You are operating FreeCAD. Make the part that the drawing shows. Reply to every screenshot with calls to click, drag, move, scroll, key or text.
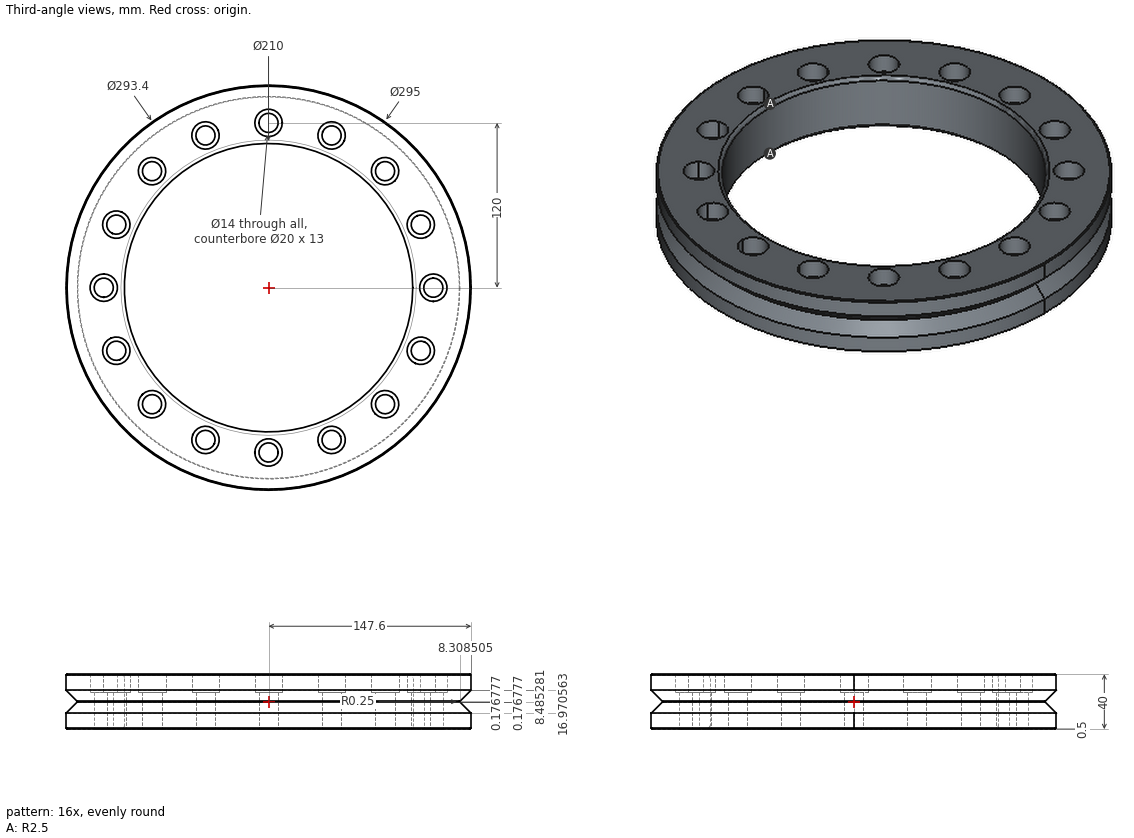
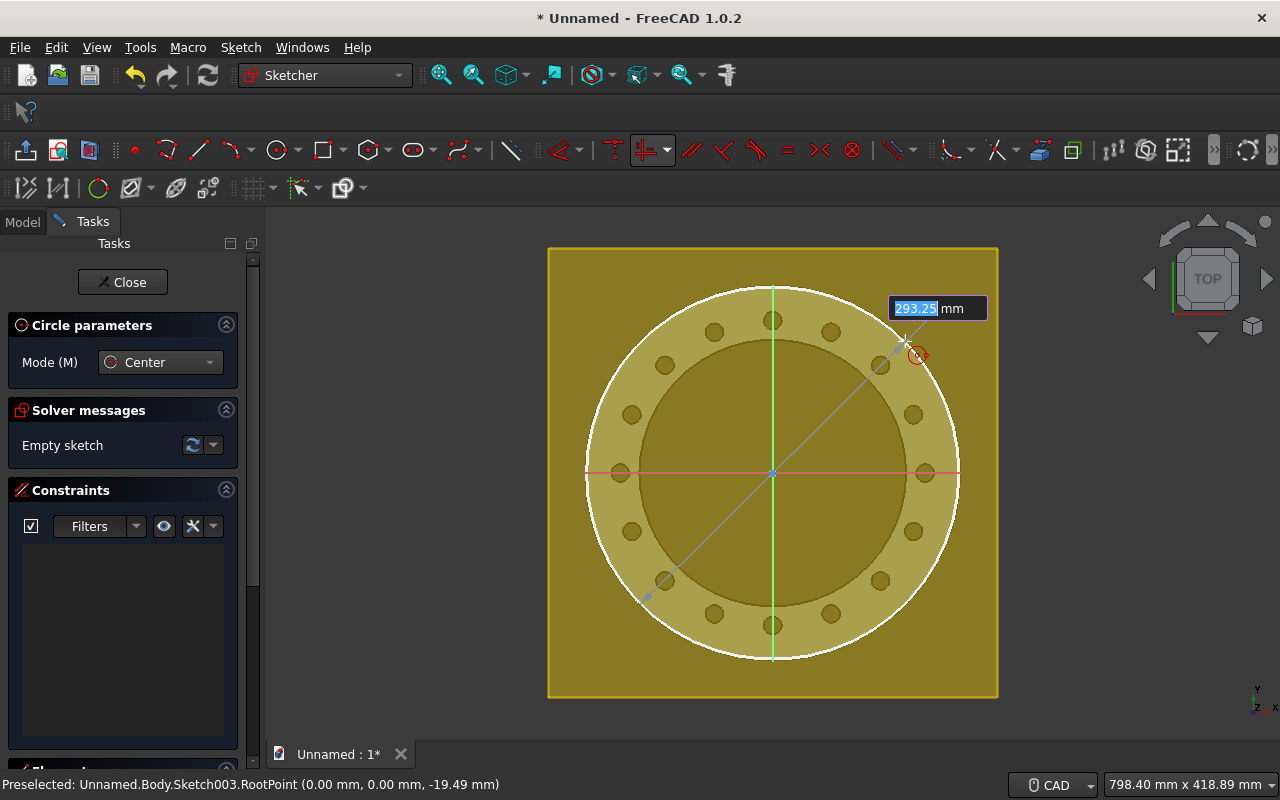
text(295)
key(Return)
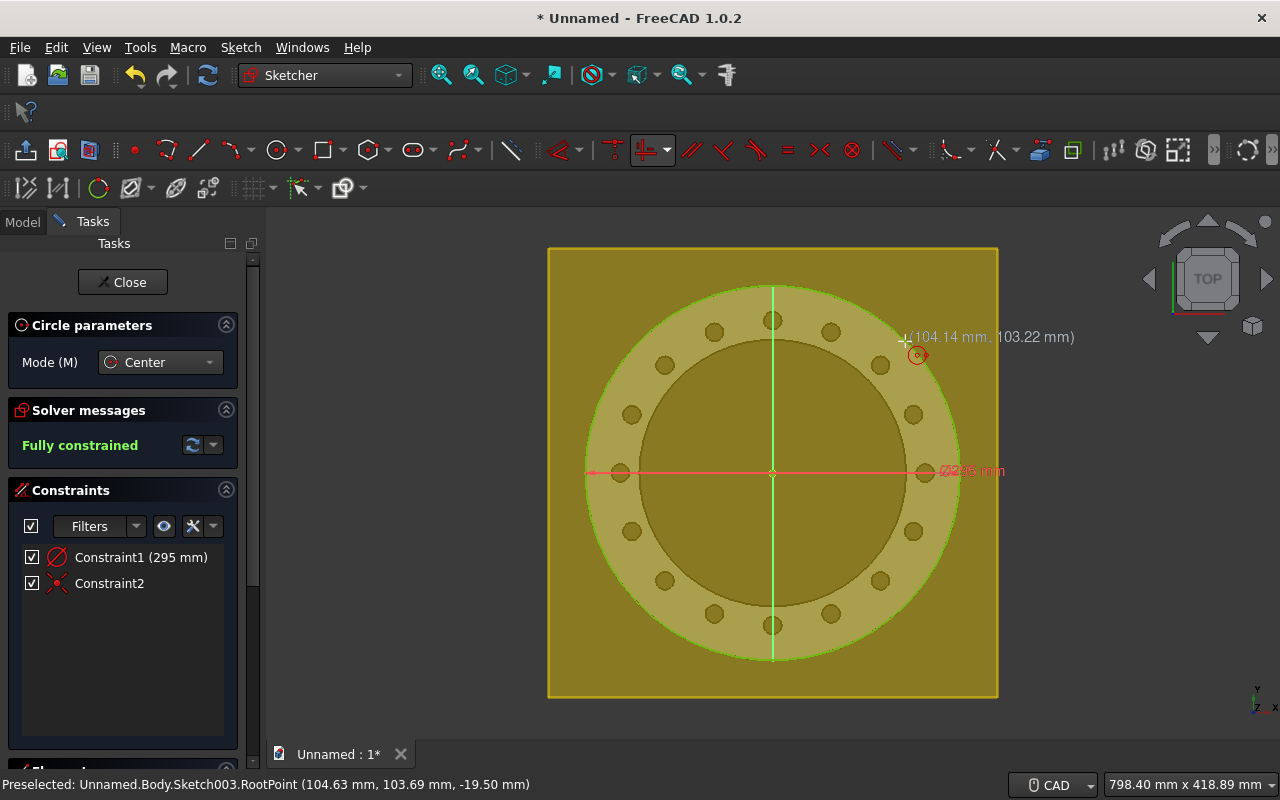
click(773, 473)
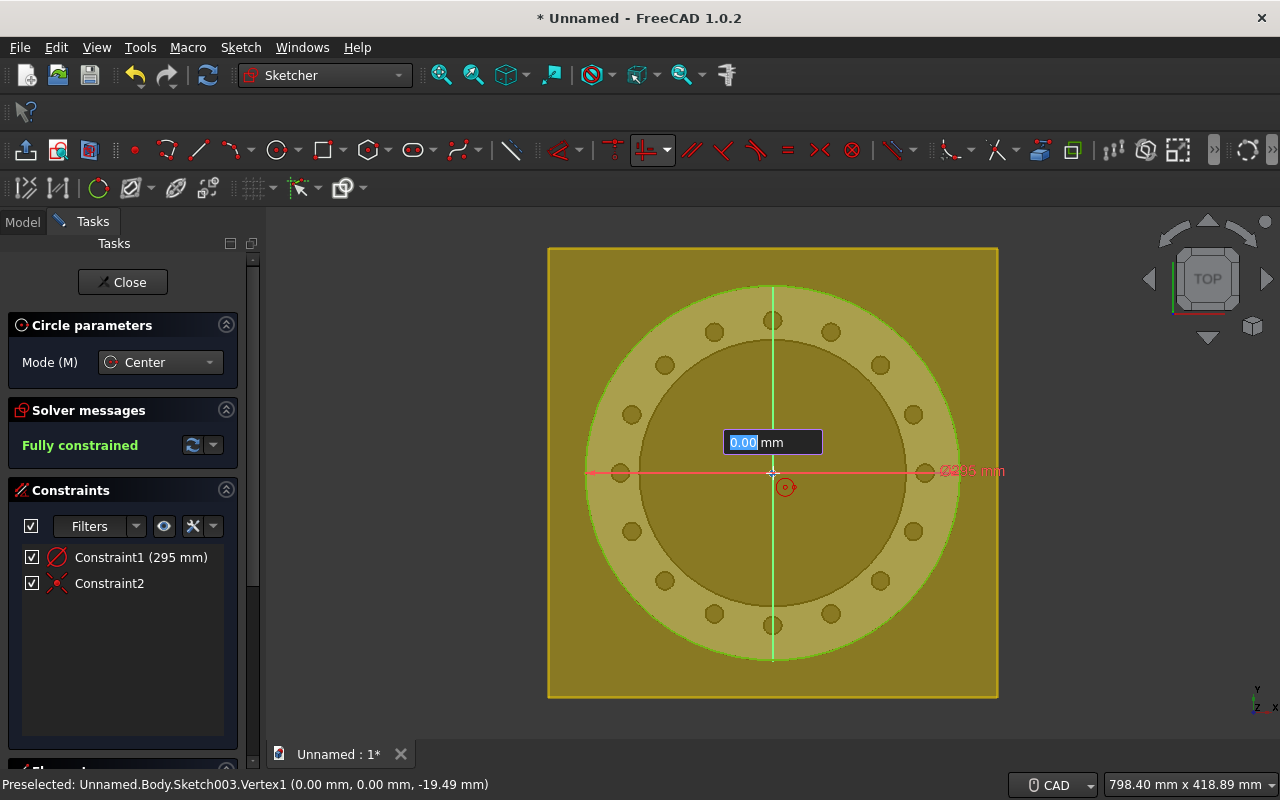
scroll(904, 341, up, 14)
move(902, 343)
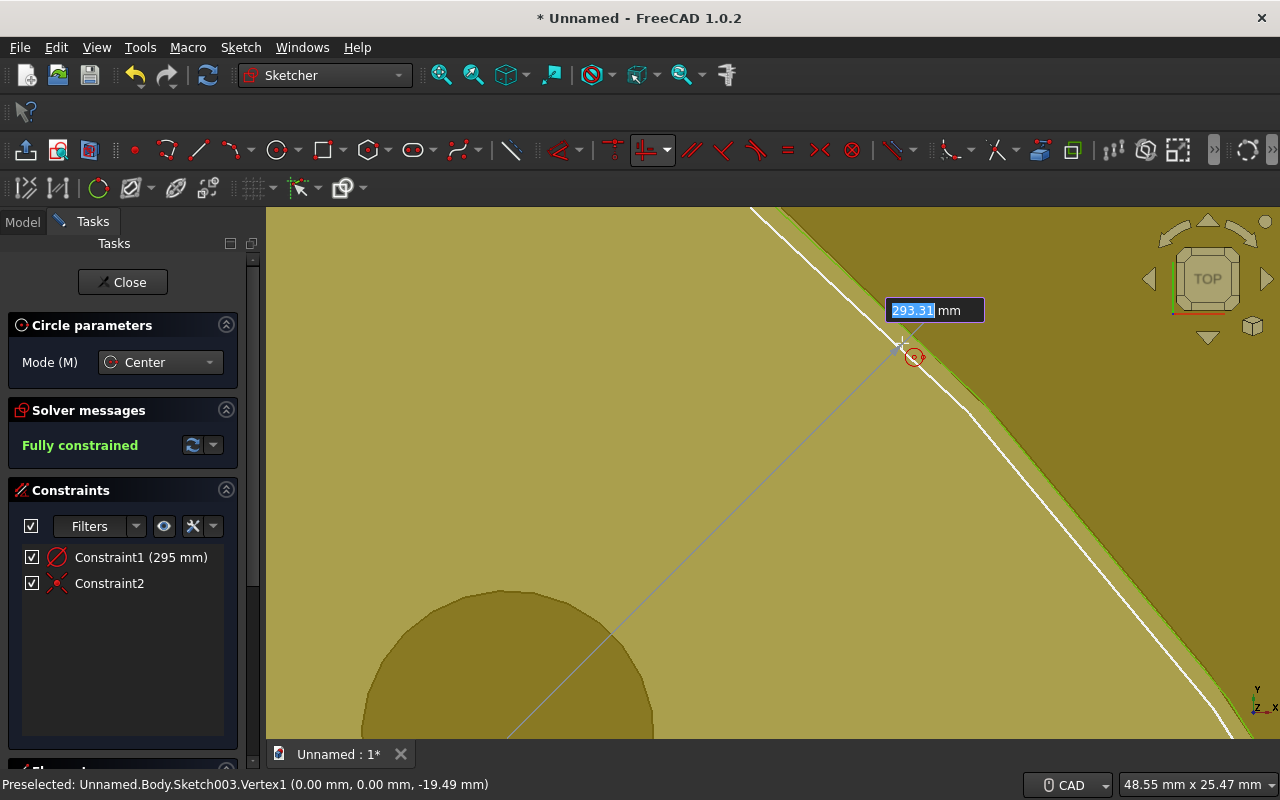
text(293.4)
key(Return)
key(Escape)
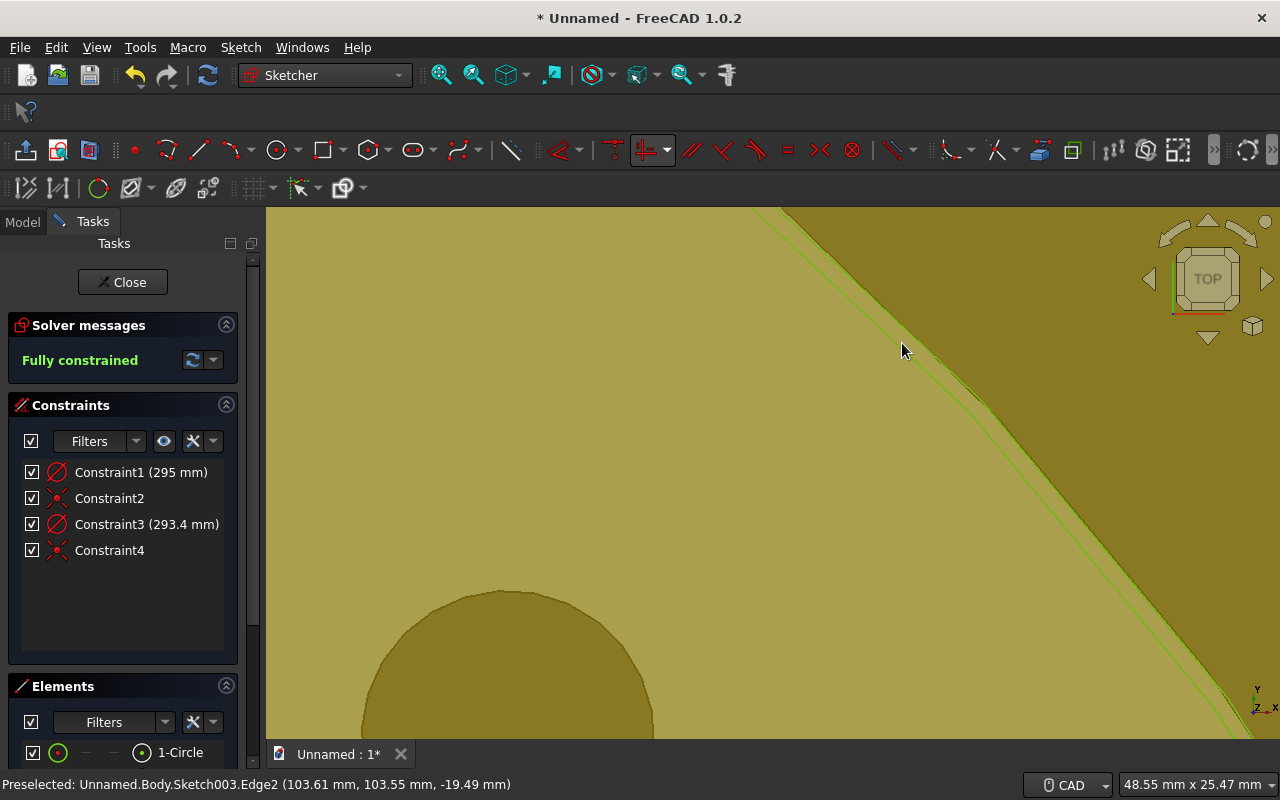
click(123, 282)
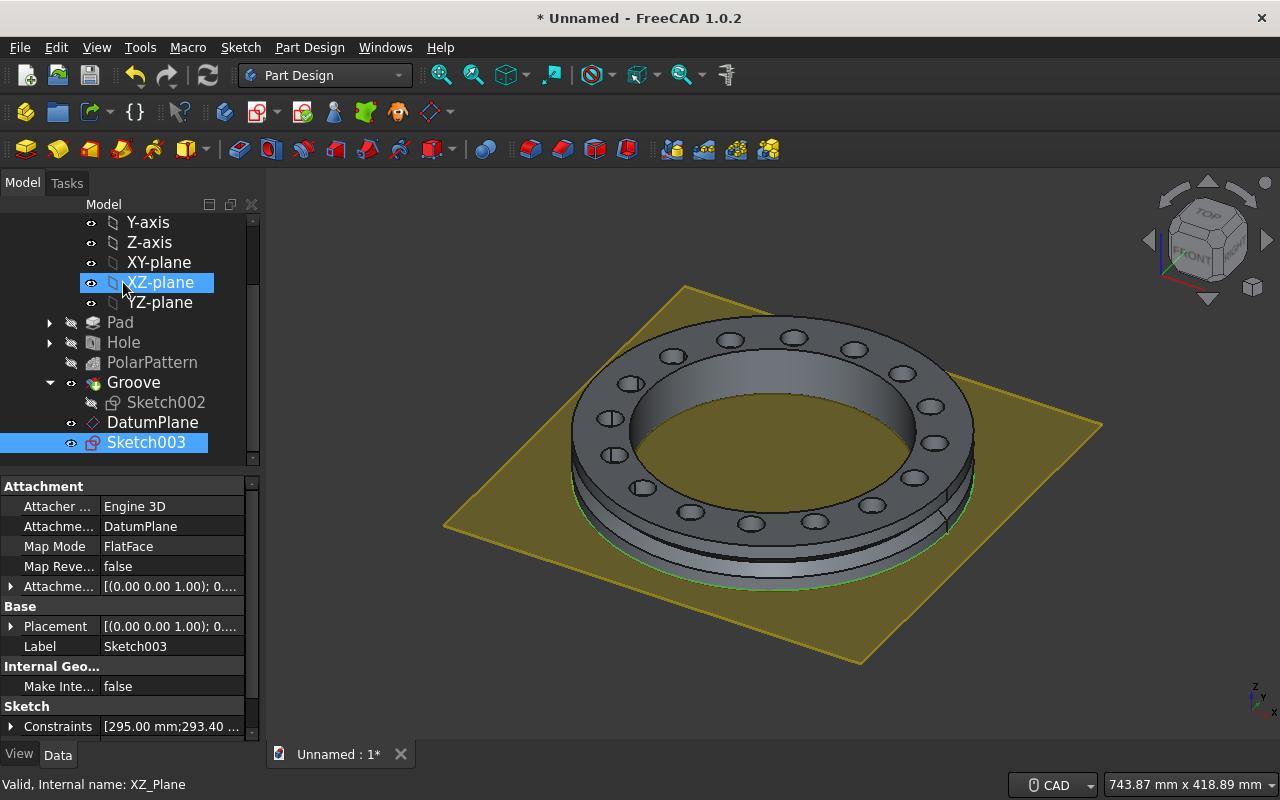
click(240, 150)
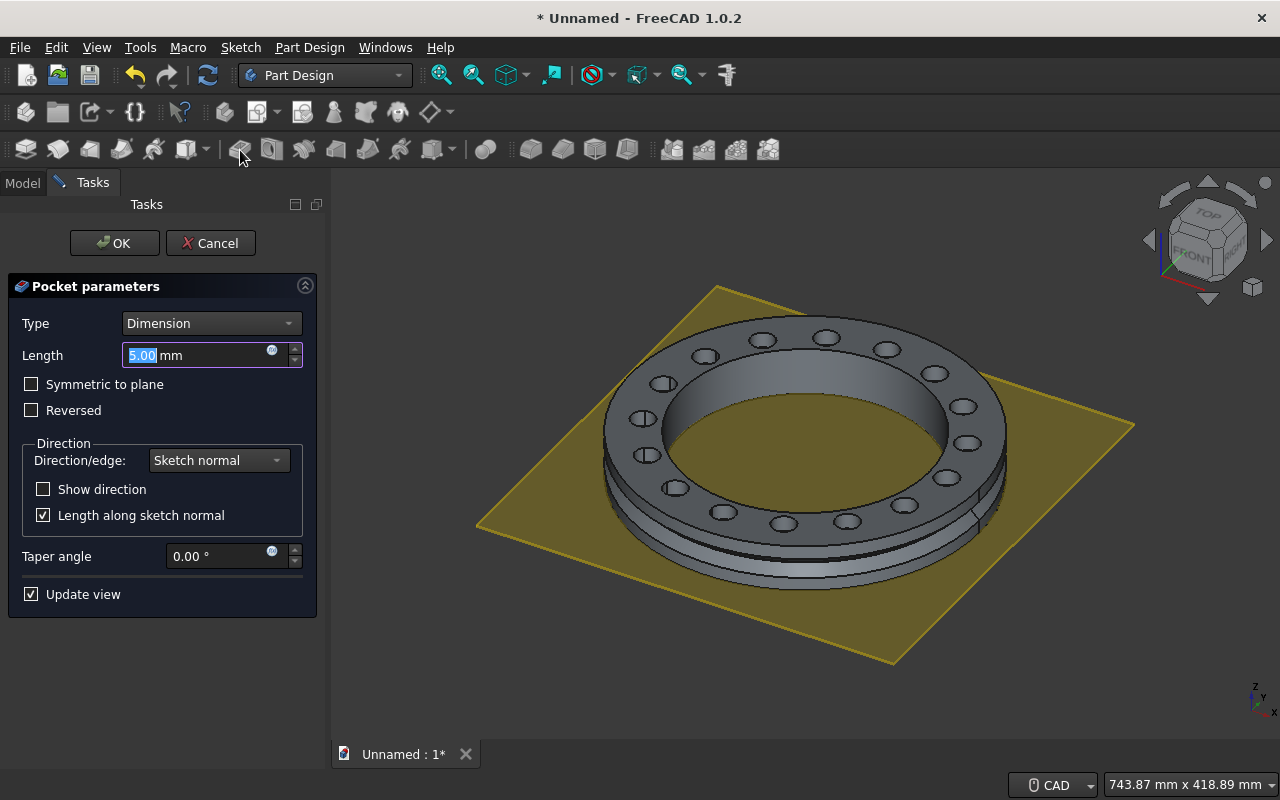
text(0.5)
key(Tab)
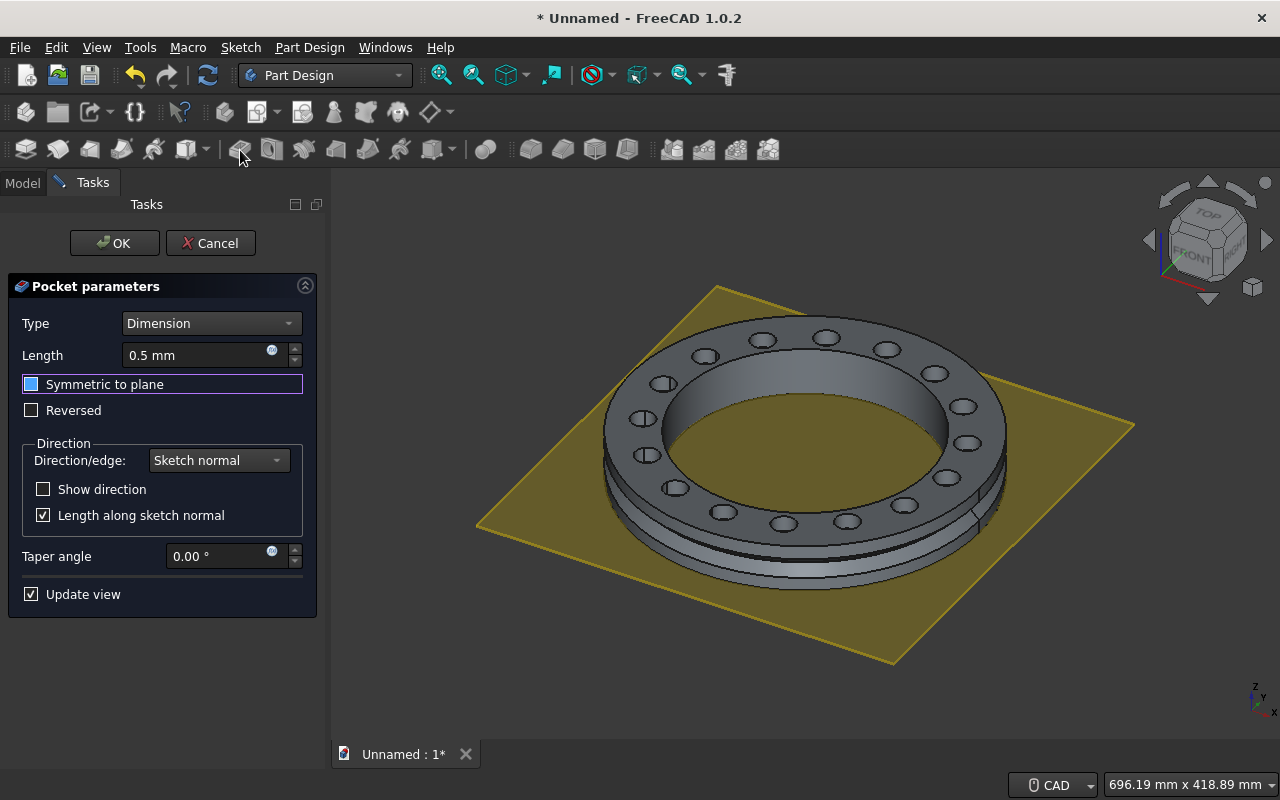
click(115, 243)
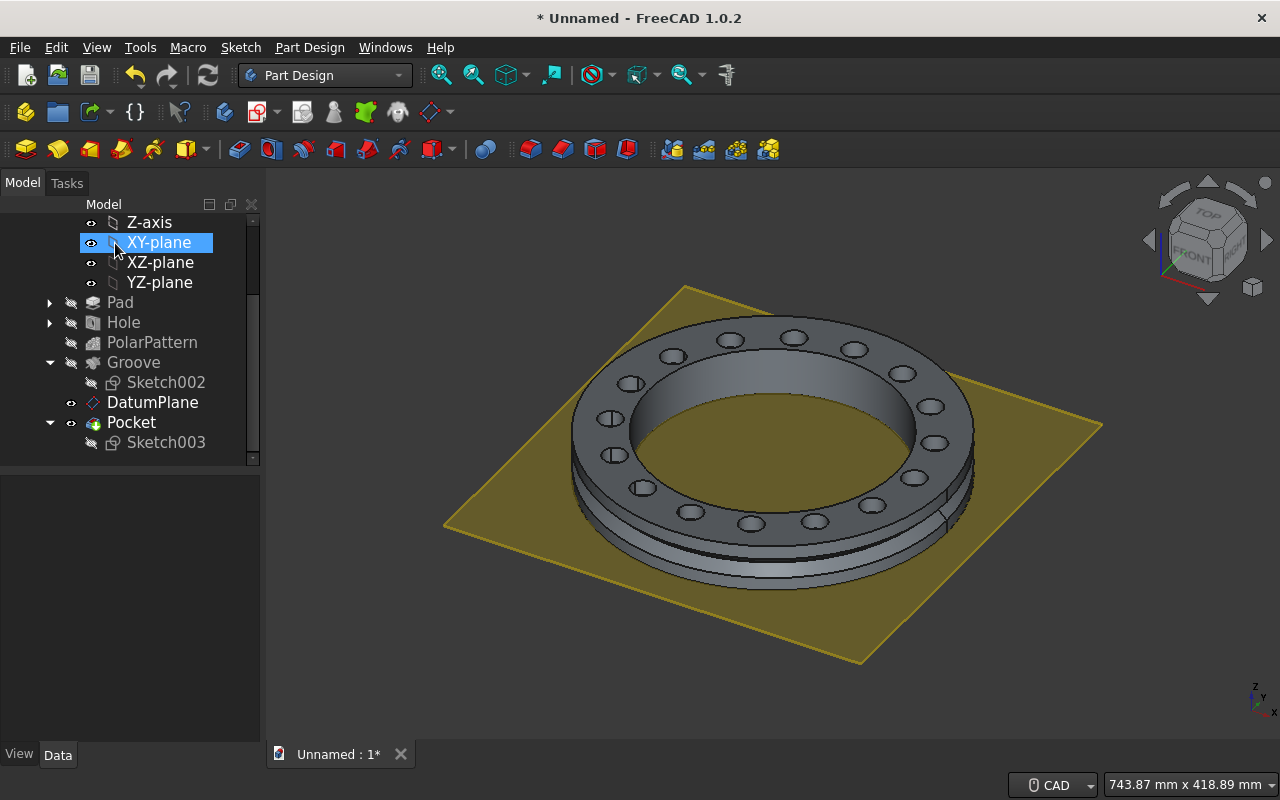
click(116, 403)
key(space)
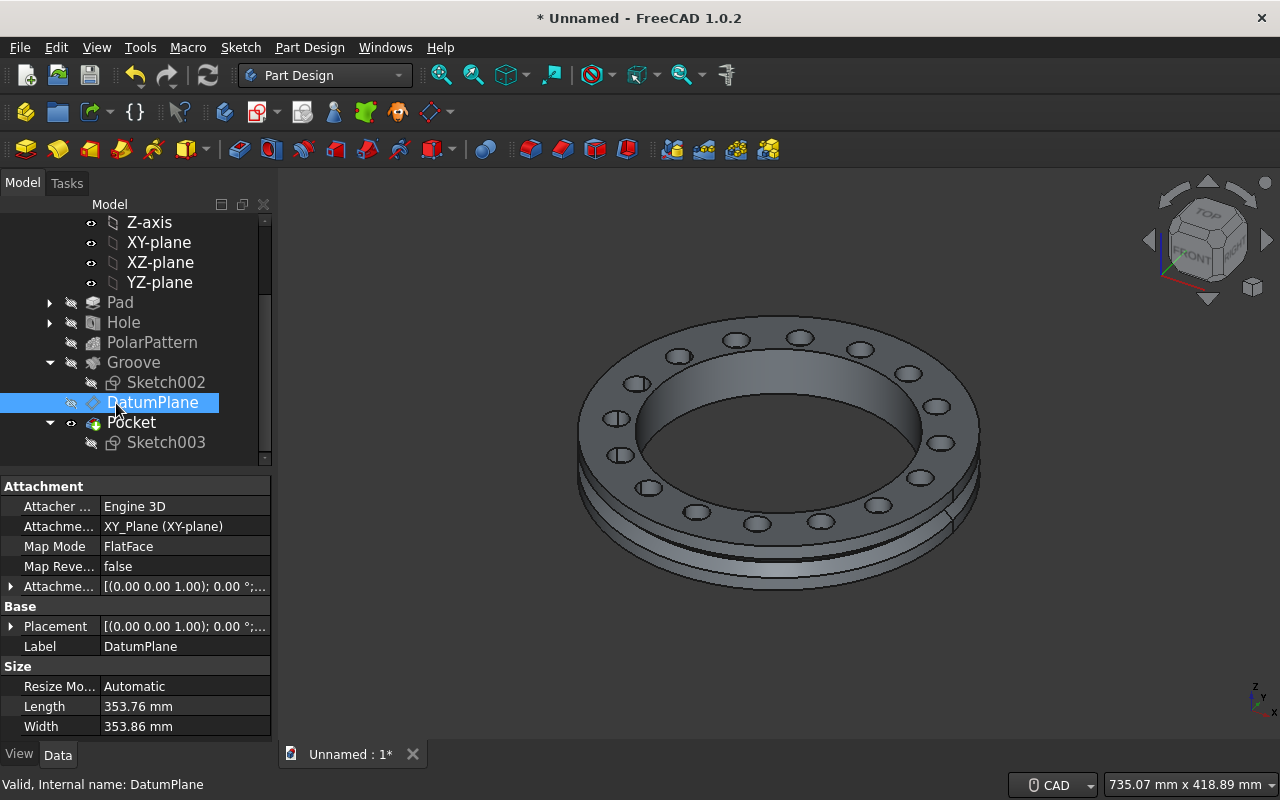
click(116, 423)